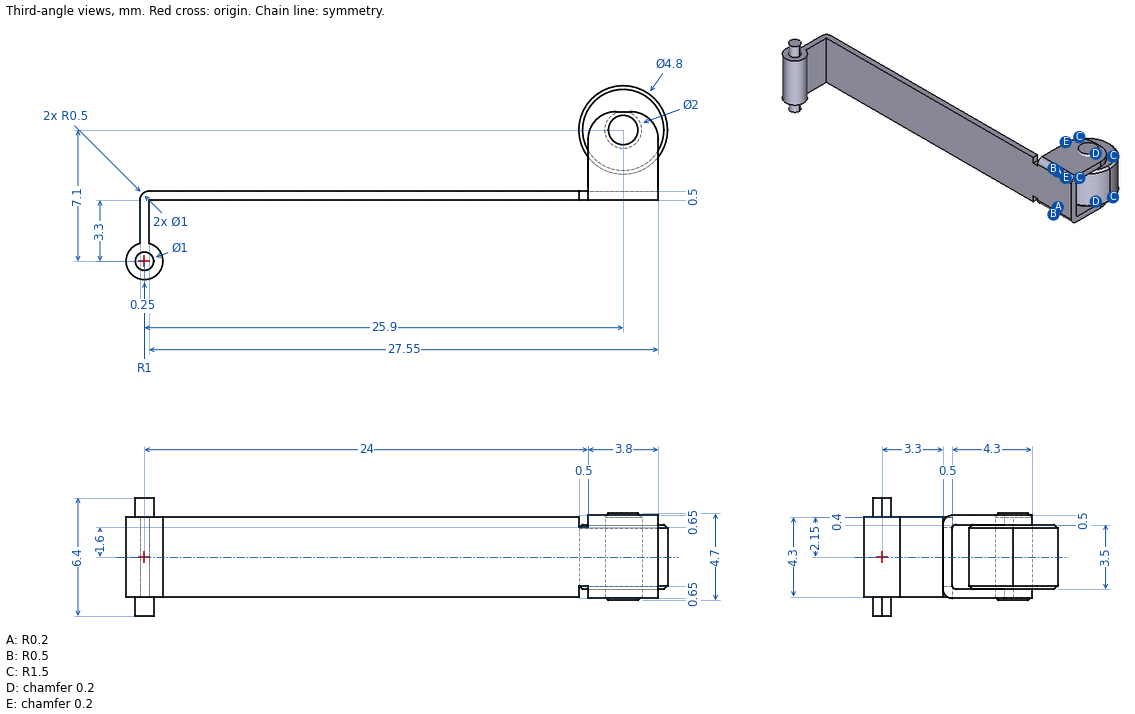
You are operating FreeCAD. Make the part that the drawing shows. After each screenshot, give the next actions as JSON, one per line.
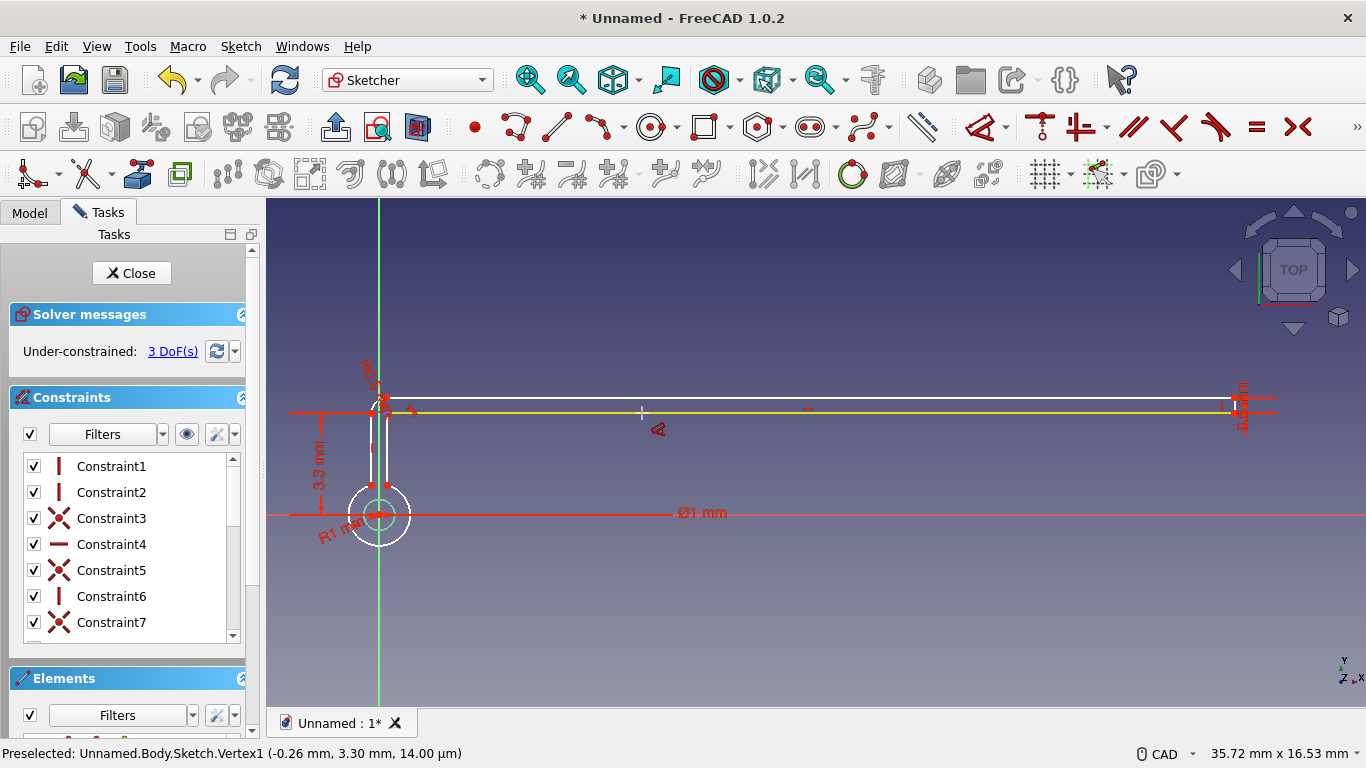
{"action": "left_click", "coordinate": [641, 413]}
{"action": "left_click", "coordinate": [794, 379]}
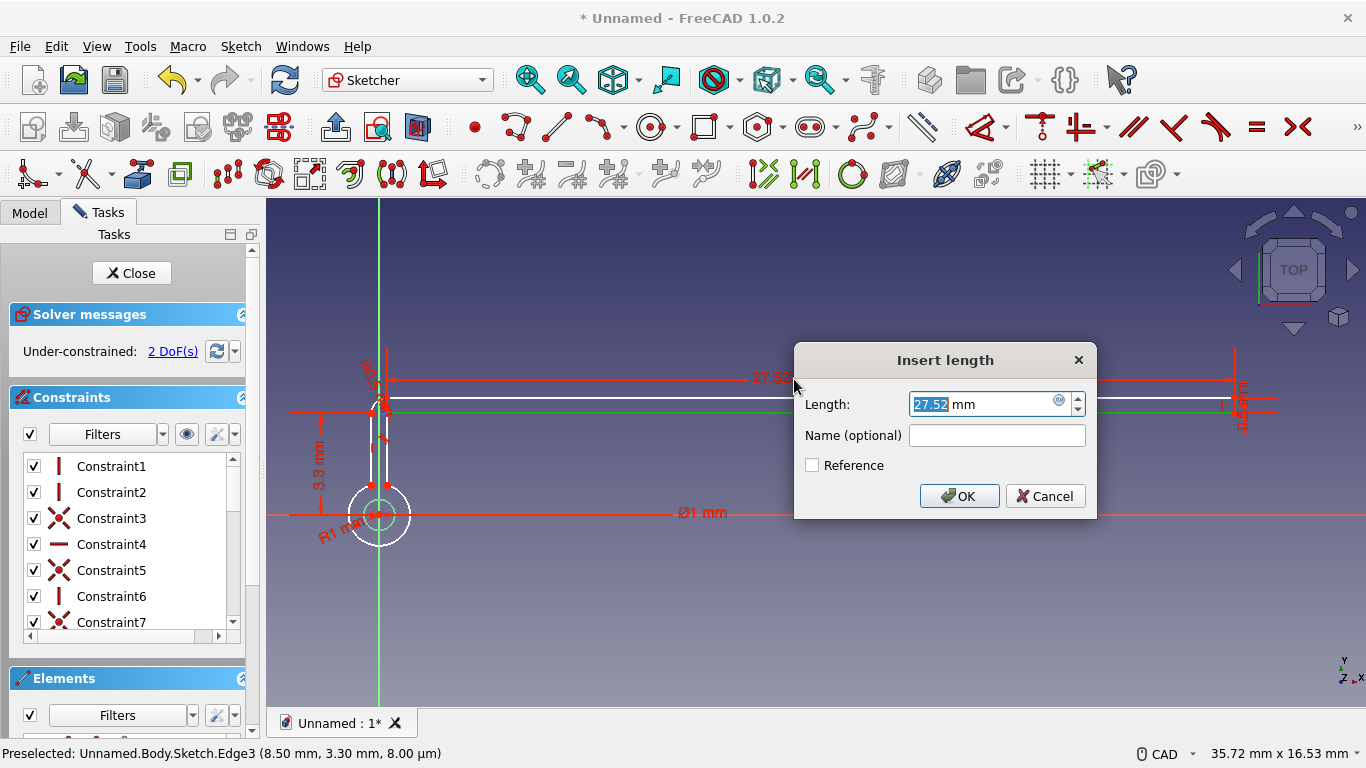
{"action": "type", "text": "27.55"}
{"action": "key", "text": "Return"}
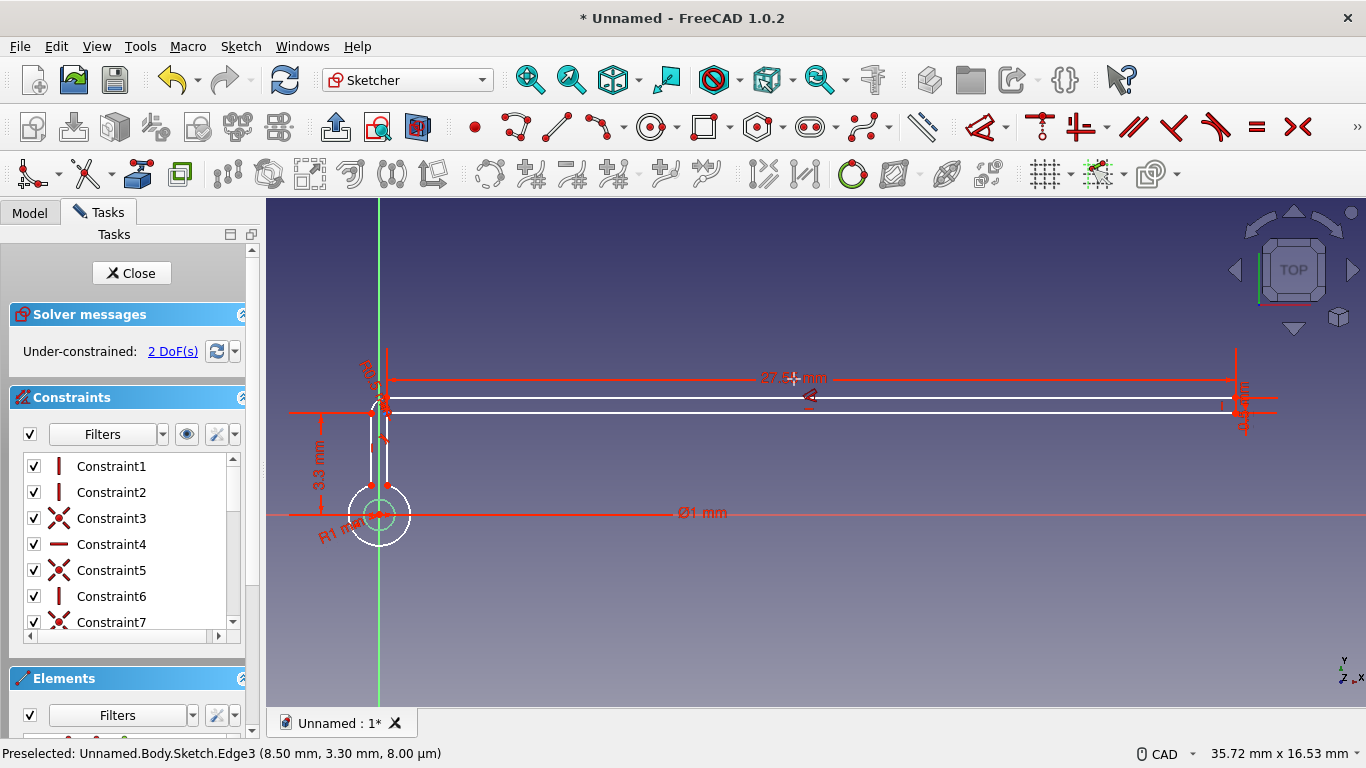
{"action": "left_click", "coordinate": [981, 398]}
{"action": "left_click", "coordinate": [607, 364]}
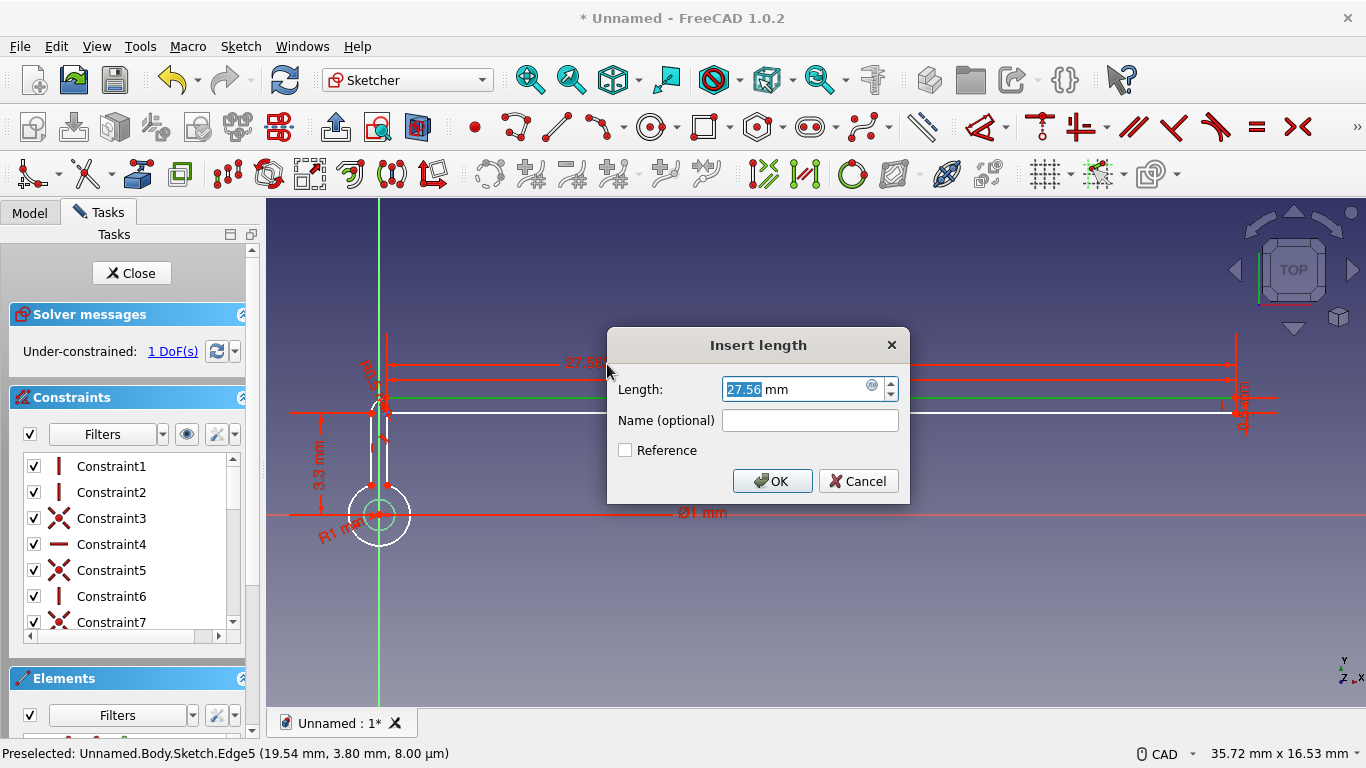
{"action": "type", "text": "27.55"}
{"action": "key", "text": "Return"}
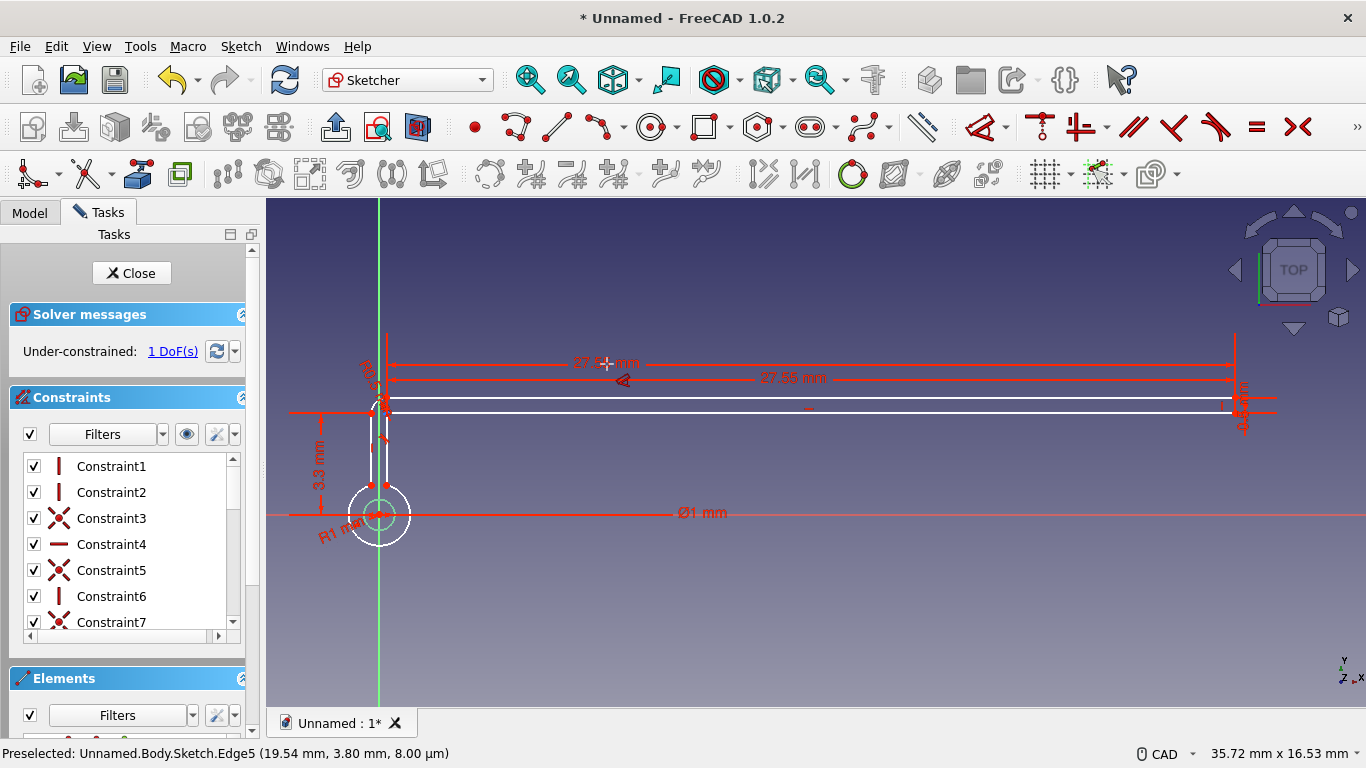
{"action": "scroll", "coordinate": [371, 413], "scroll_direction": "up", "scroll_amount": 9}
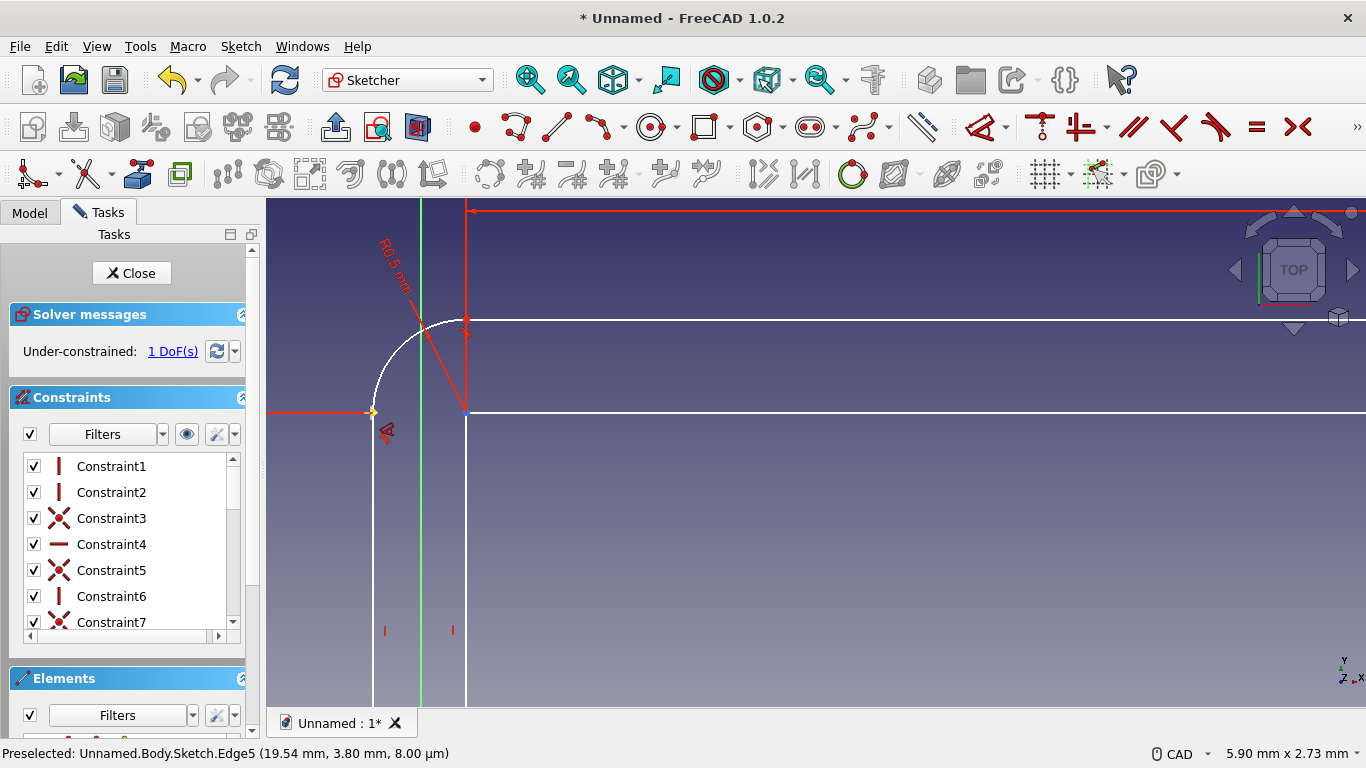
{"action": "left_click", "coordinate": [373, 413]}
{"action": "left_click", "coordinate": [397, 379]}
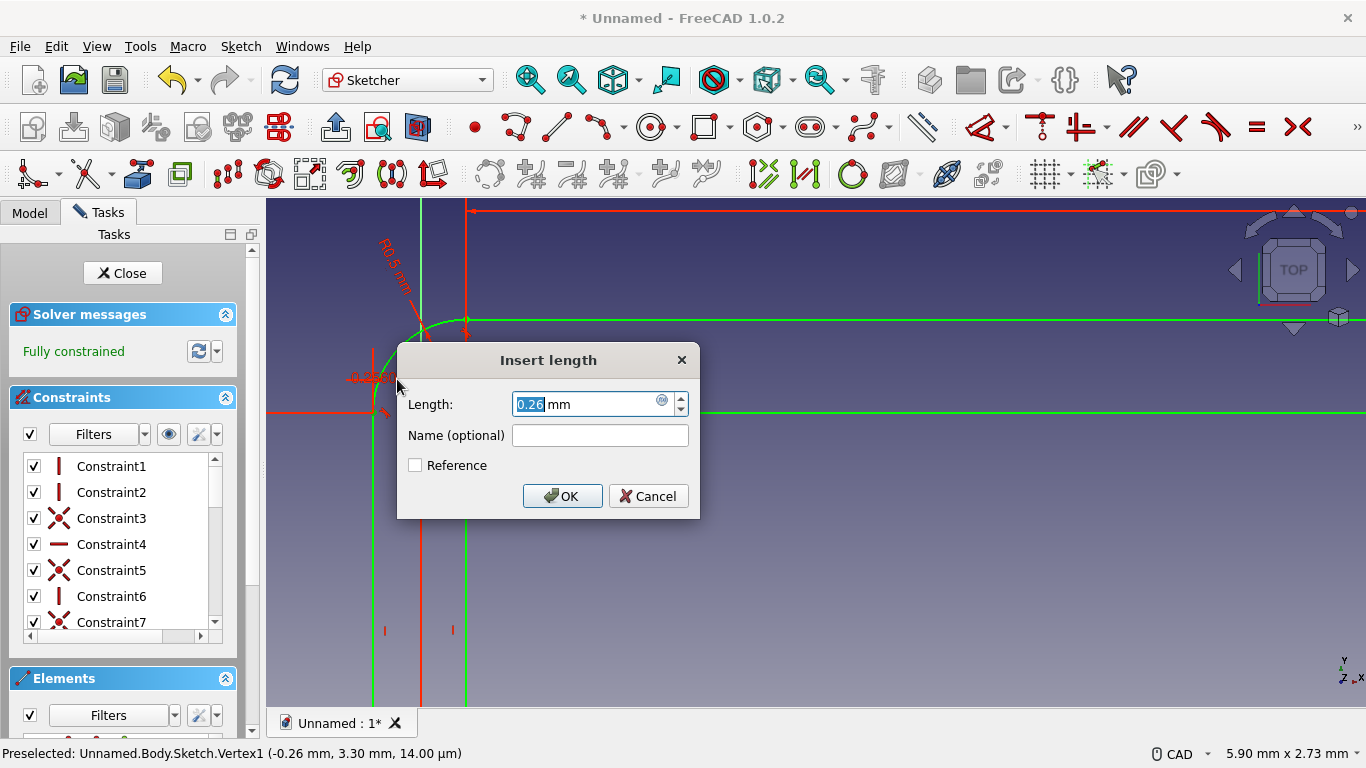
{"action": "type", "text": "0.25"}
{"action": "key", "text": "Return"}
{"action": "key", "text": "Escape"}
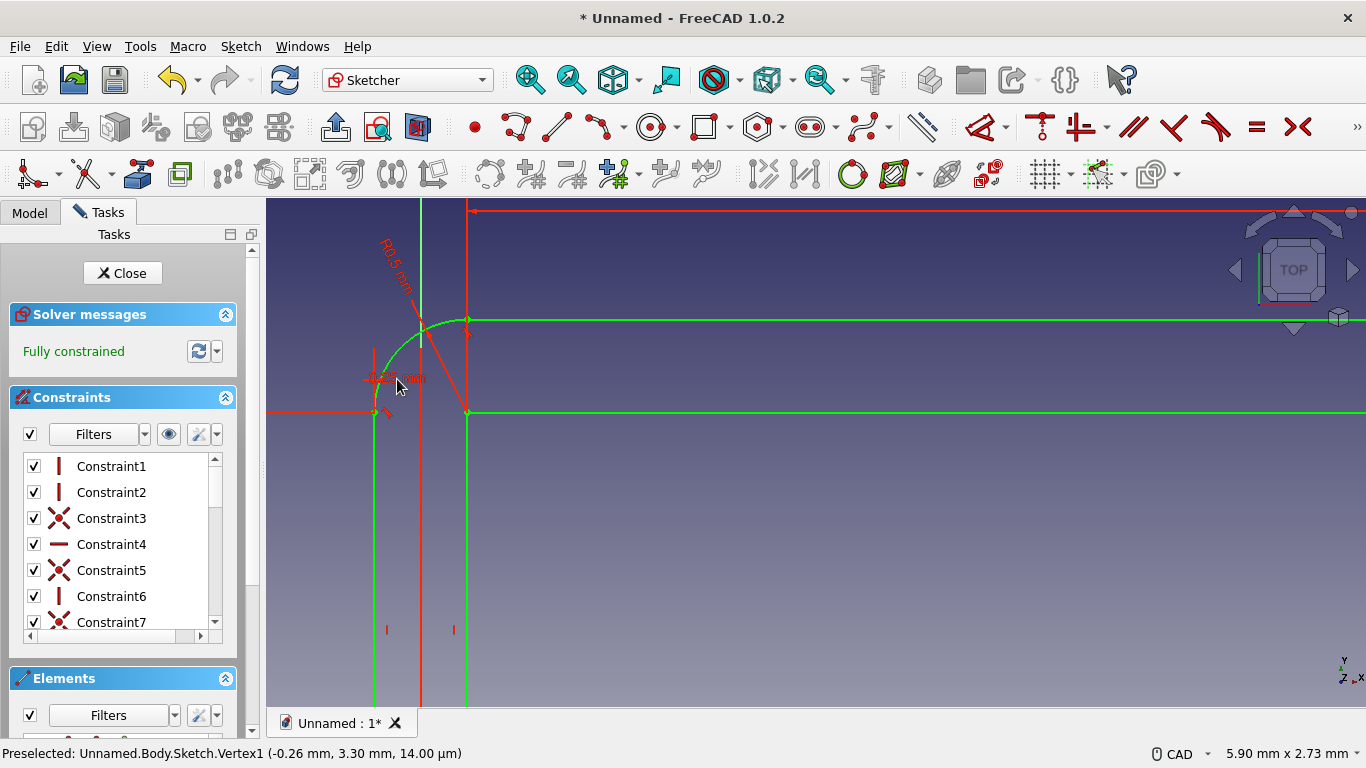
{"action": "left_click", "coordinate": [123, 273]}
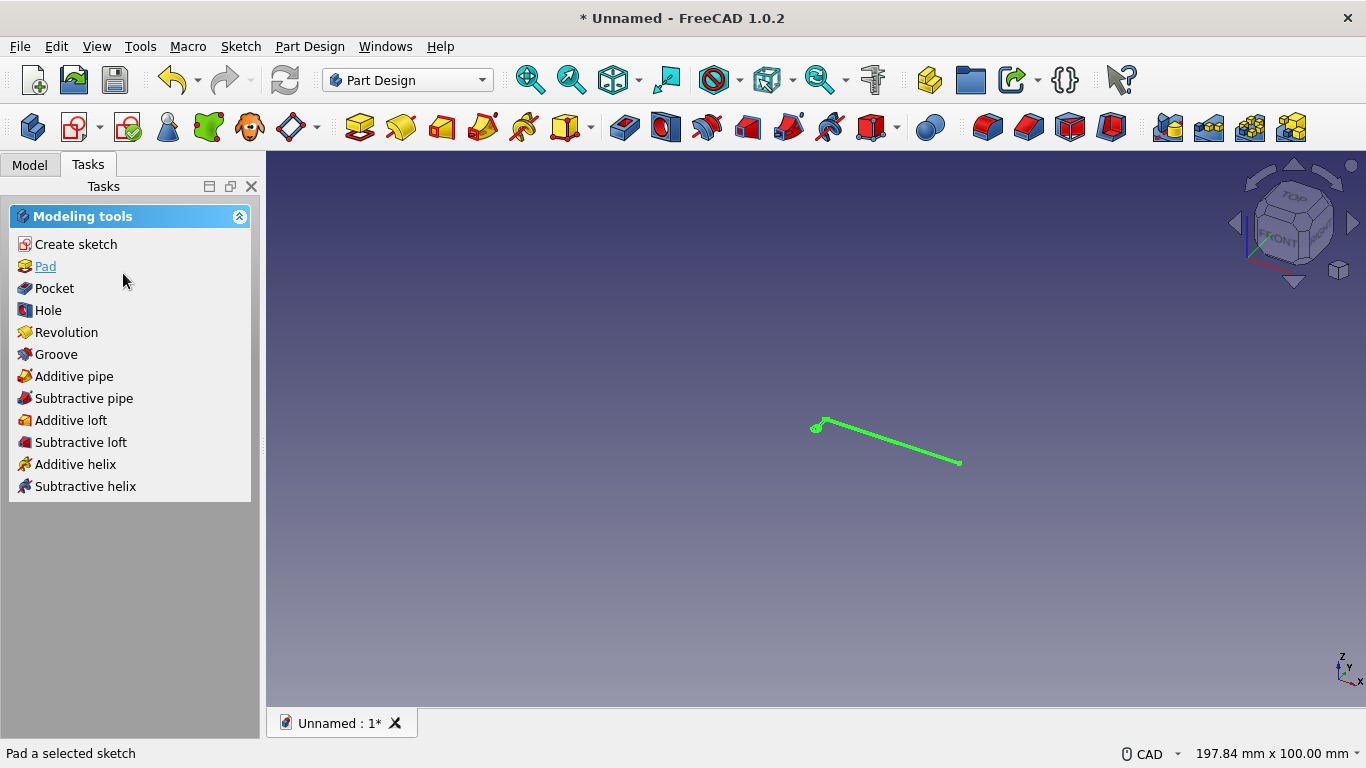
{"action": "left_click", "coordinate": [360, 128]}